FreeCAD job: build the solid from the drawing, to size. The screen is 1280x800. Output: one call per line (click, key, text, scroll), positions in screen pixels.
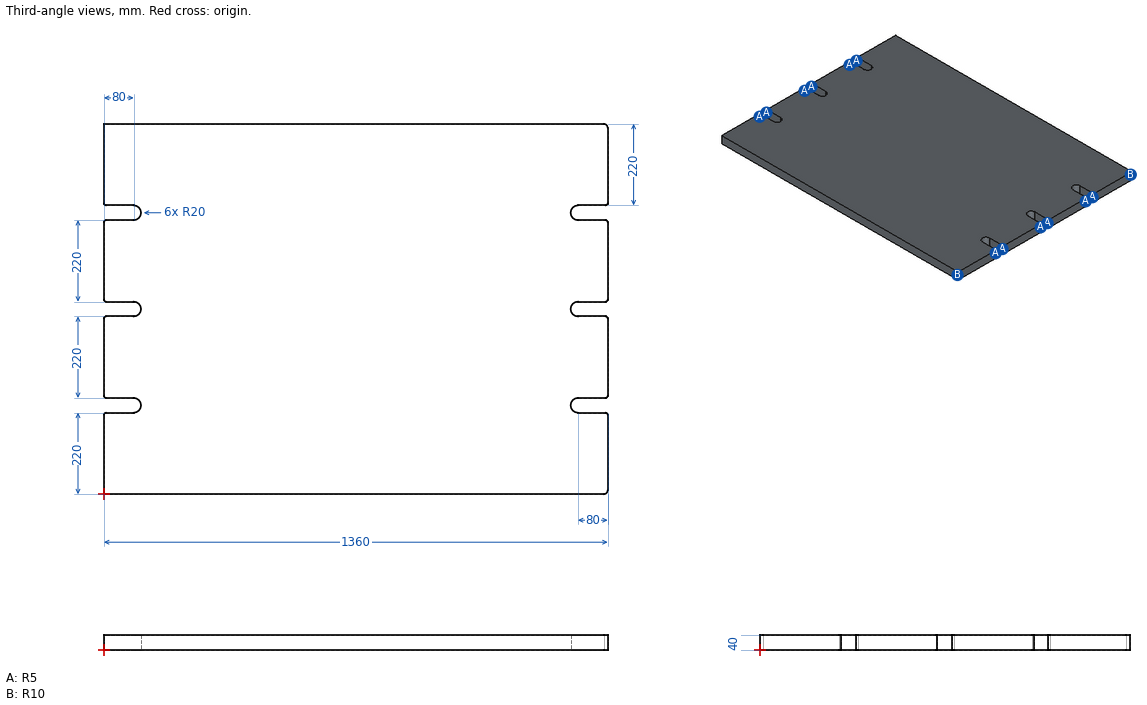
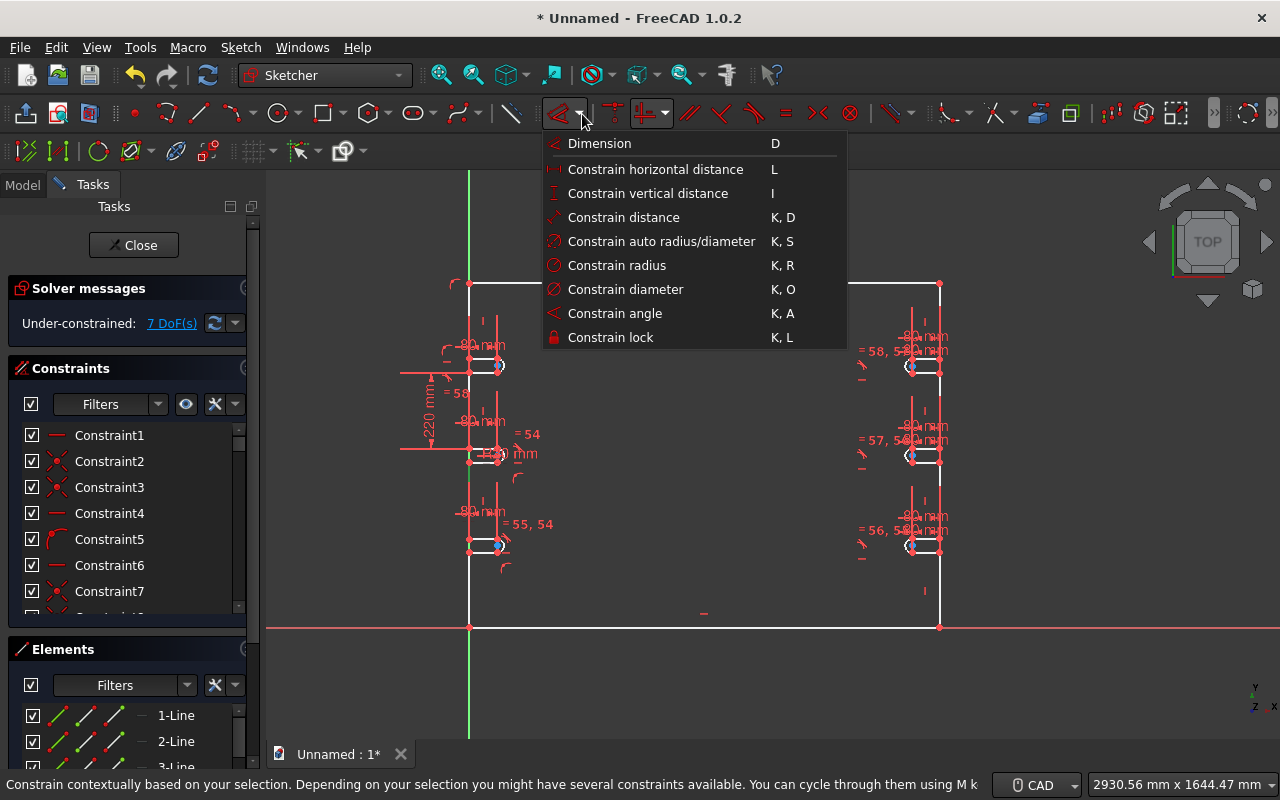
click(695, 193)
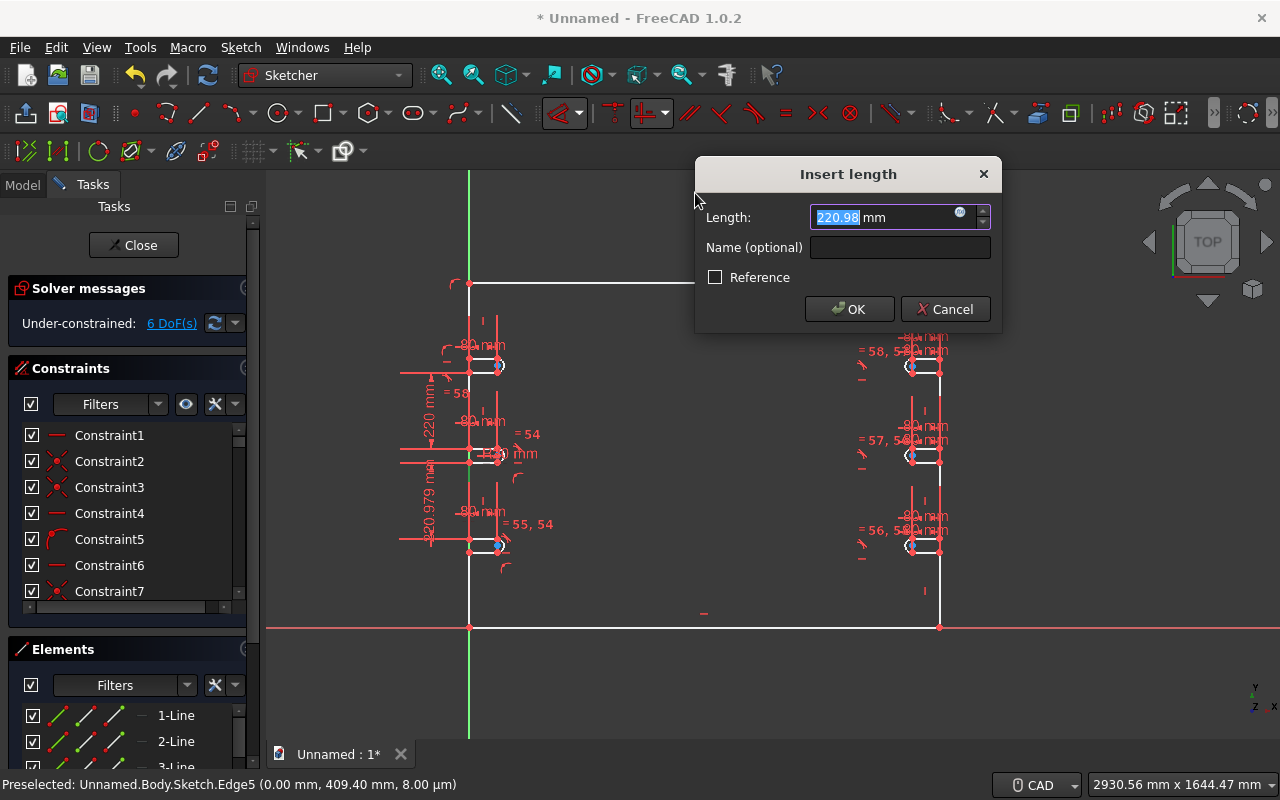
text(220)
key(Return)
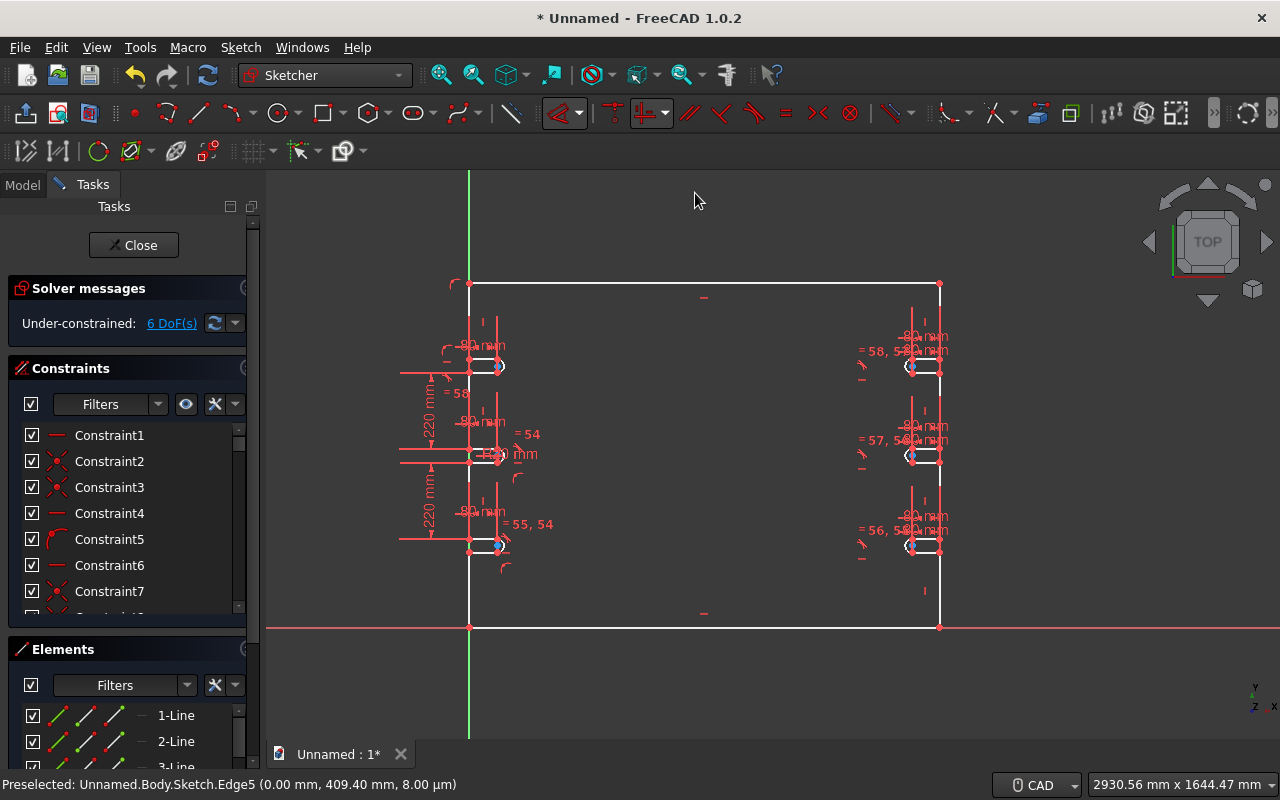
click(469, 575)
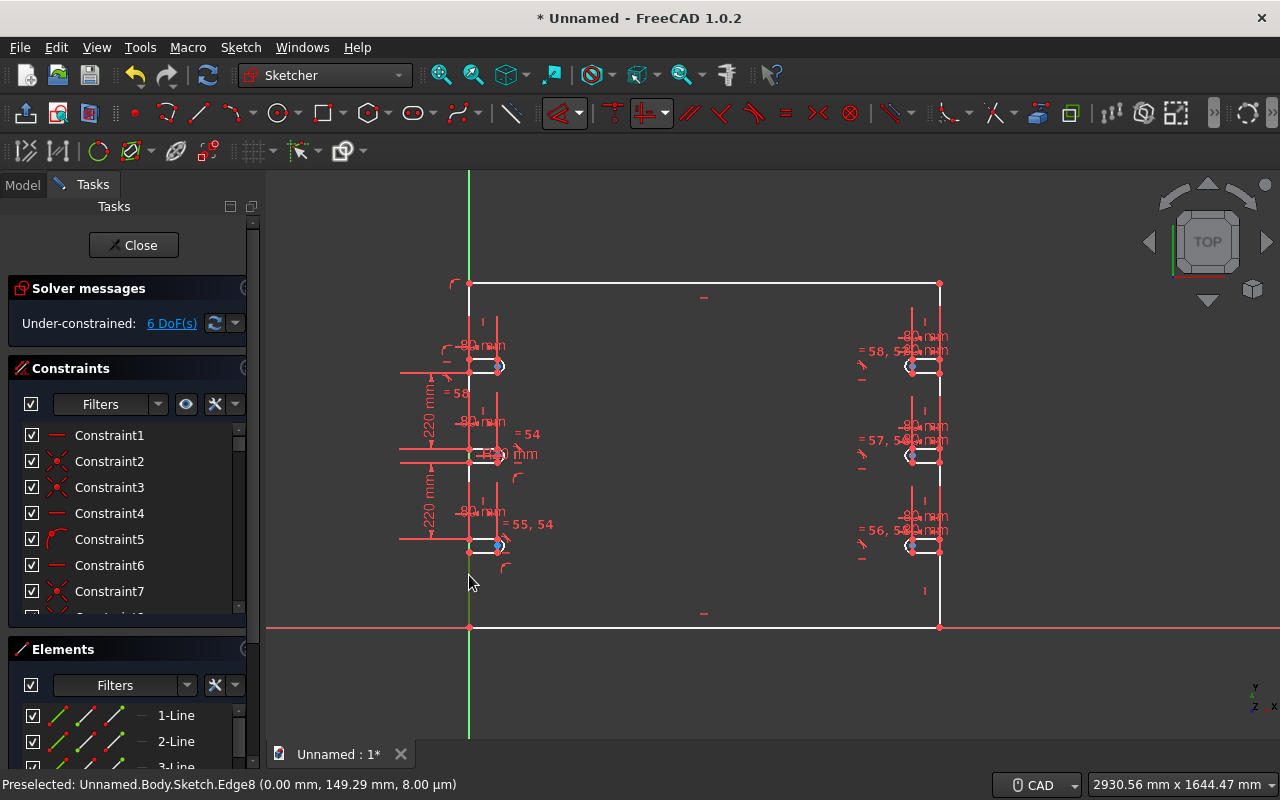
click(582, 114)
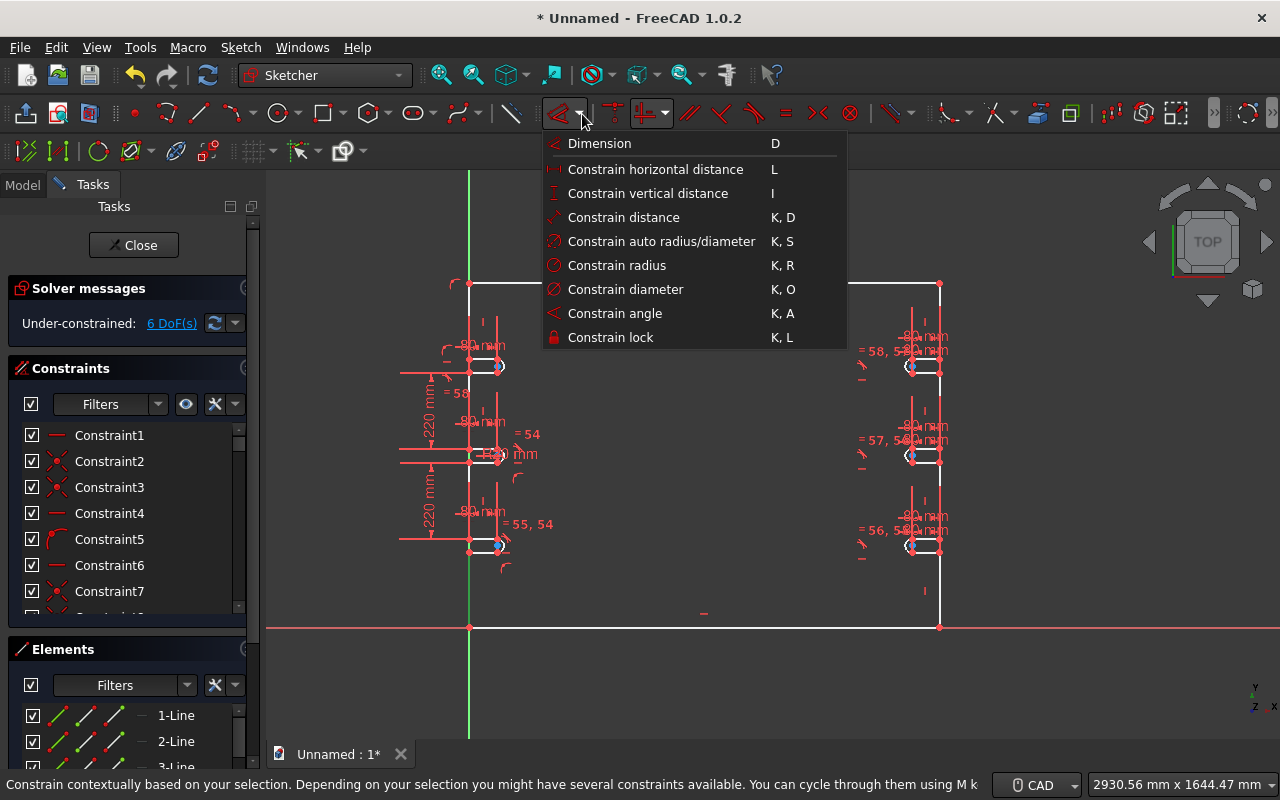
click(695, 193)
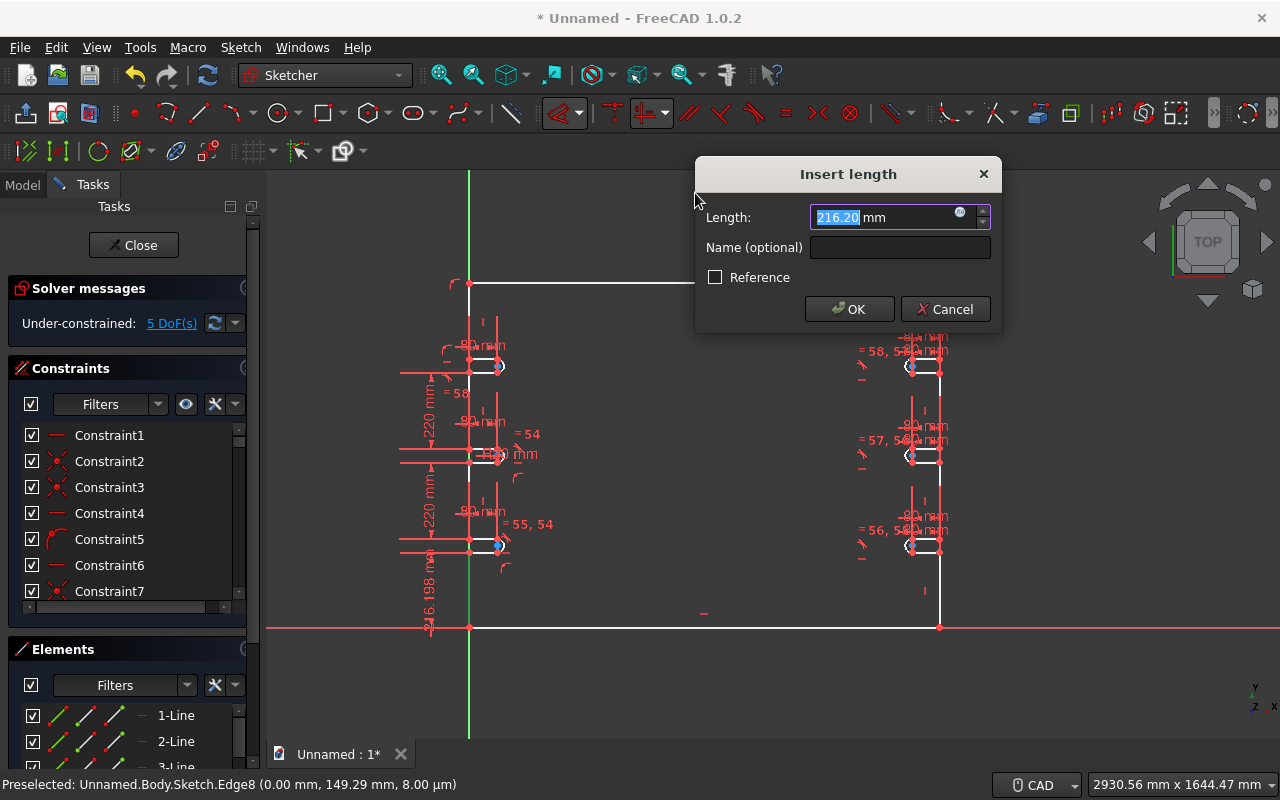
text(220)
key(Return)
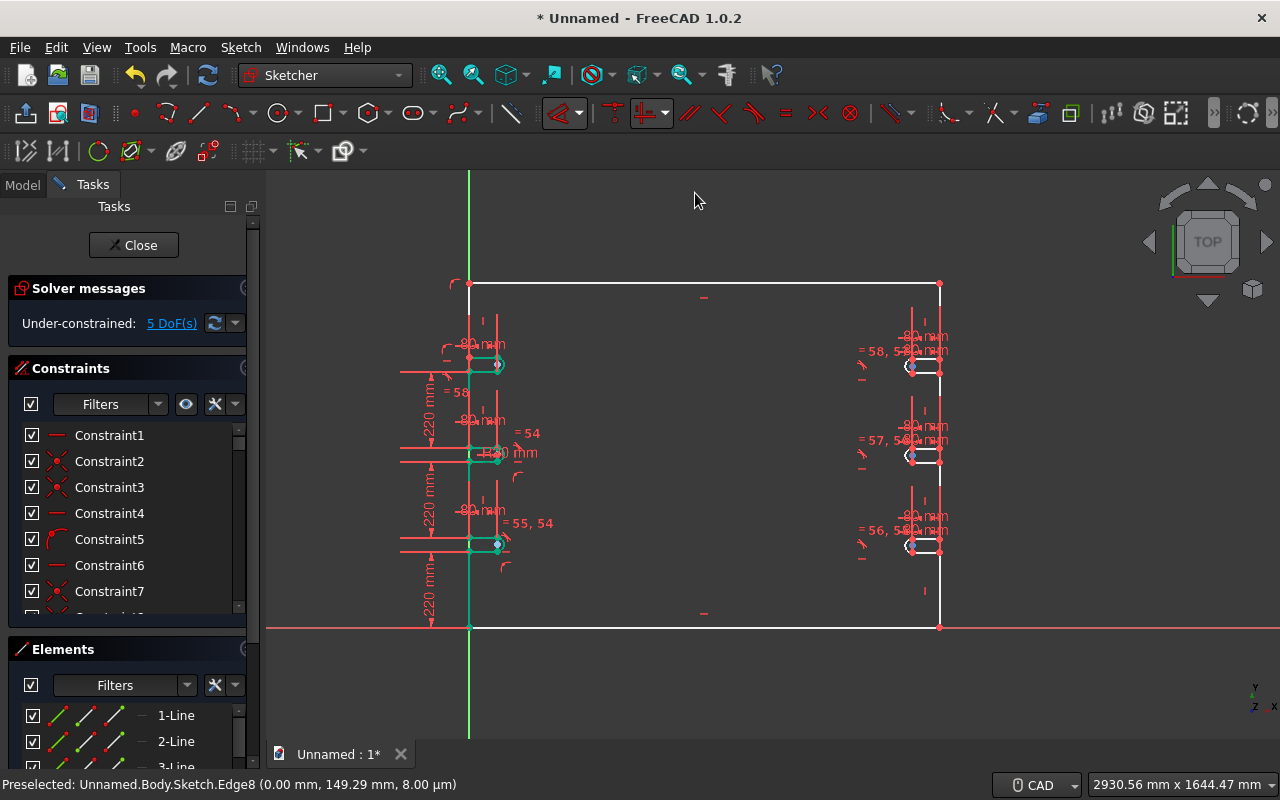
click(940, 605)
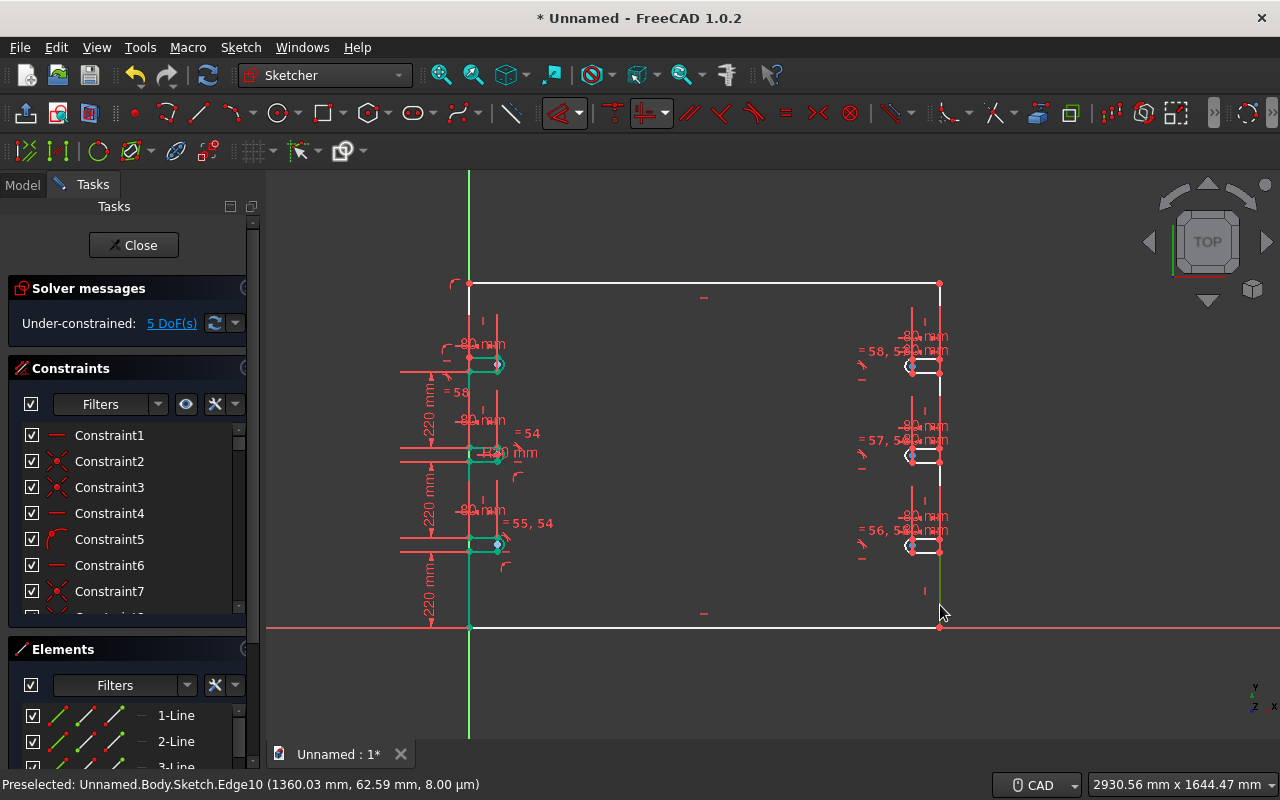
click(582, 114)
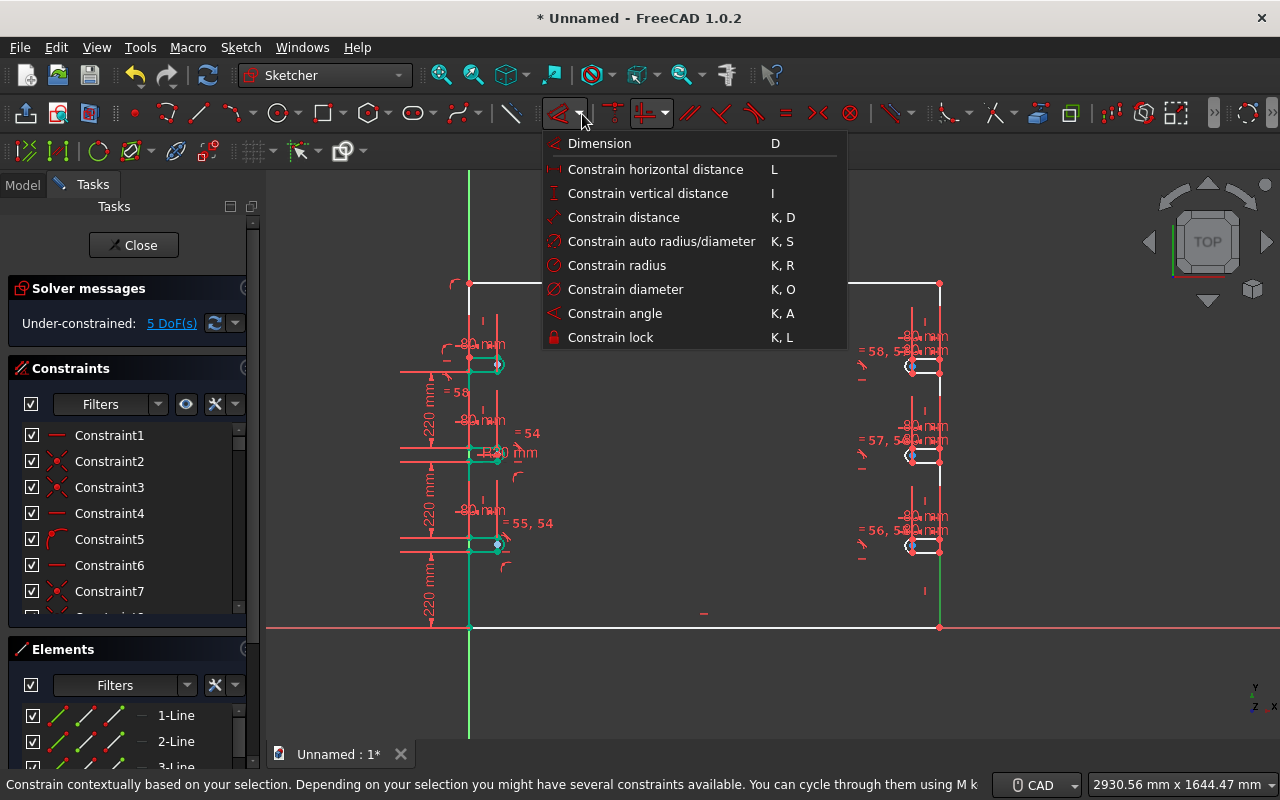
click(695, 193)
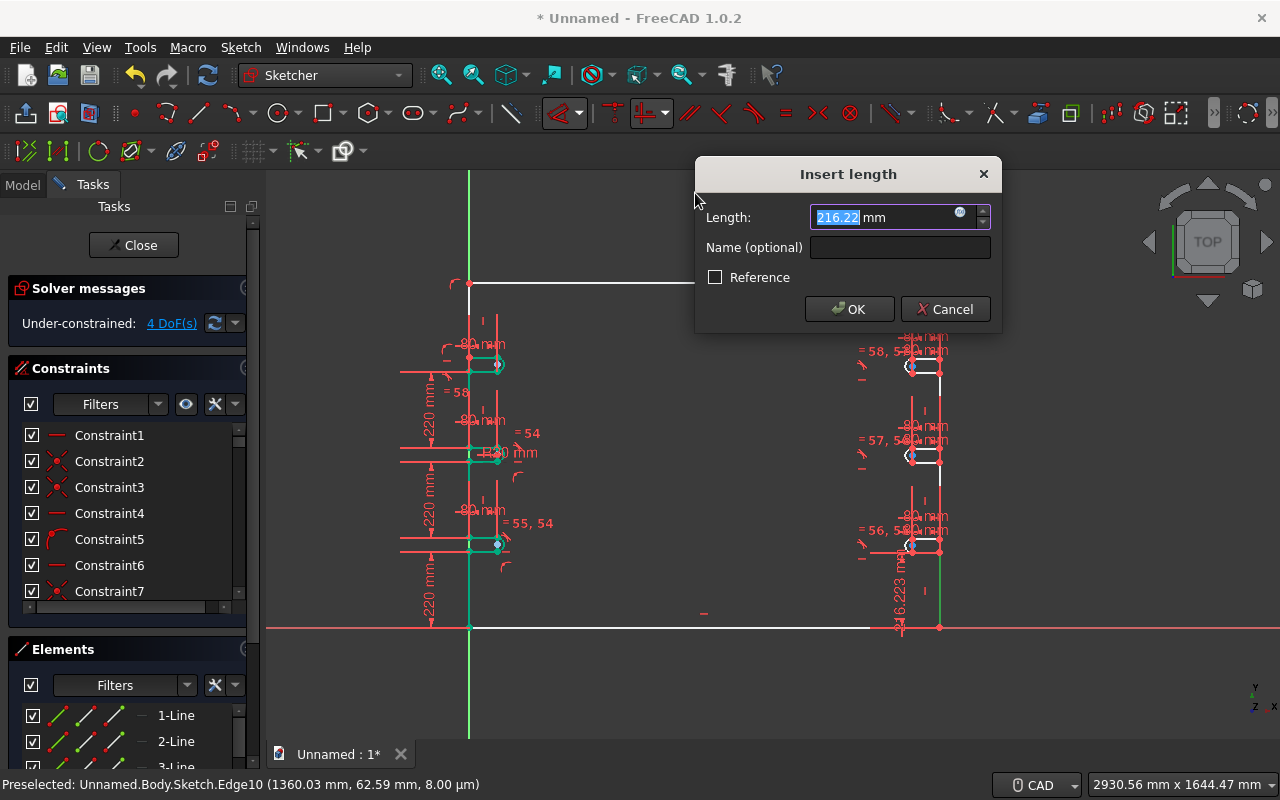
text(220)
key(Return)